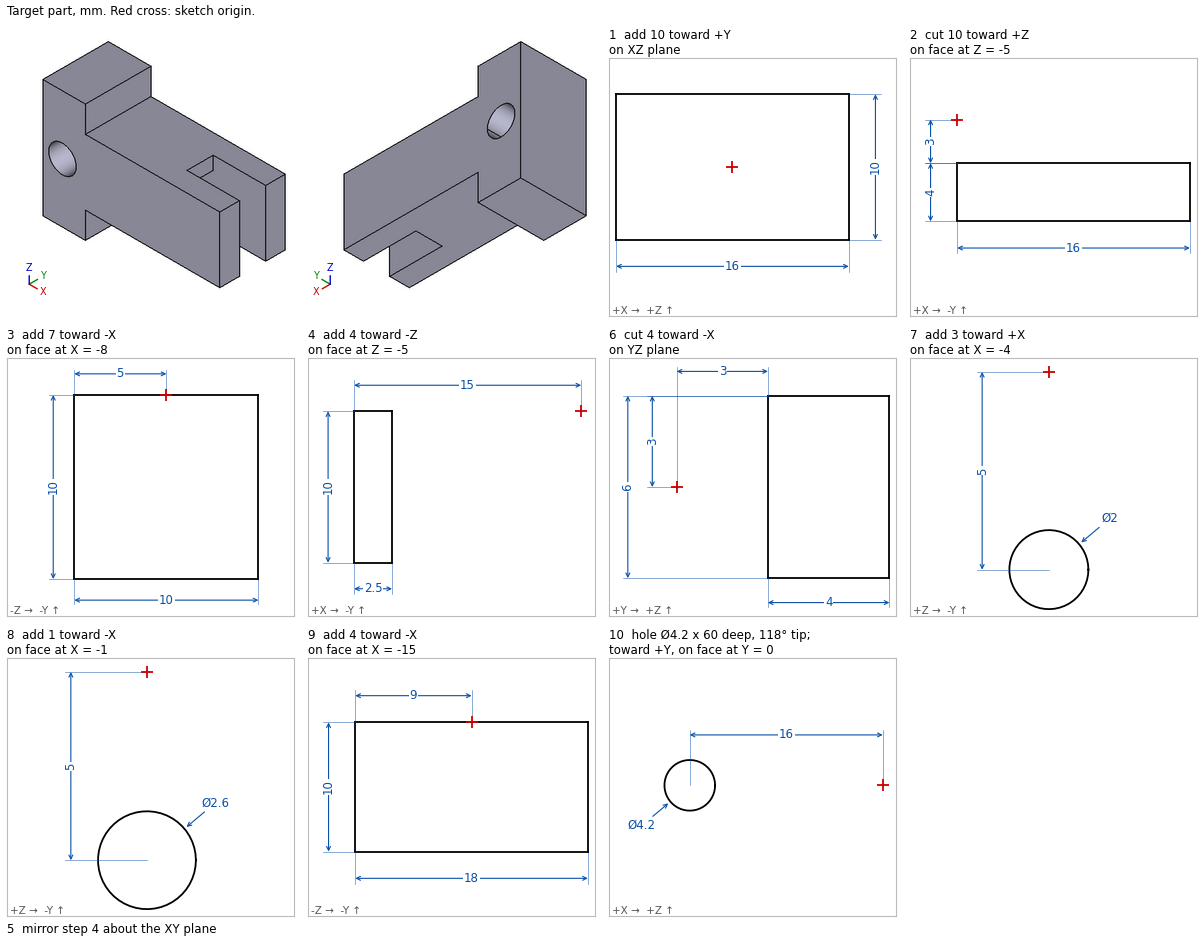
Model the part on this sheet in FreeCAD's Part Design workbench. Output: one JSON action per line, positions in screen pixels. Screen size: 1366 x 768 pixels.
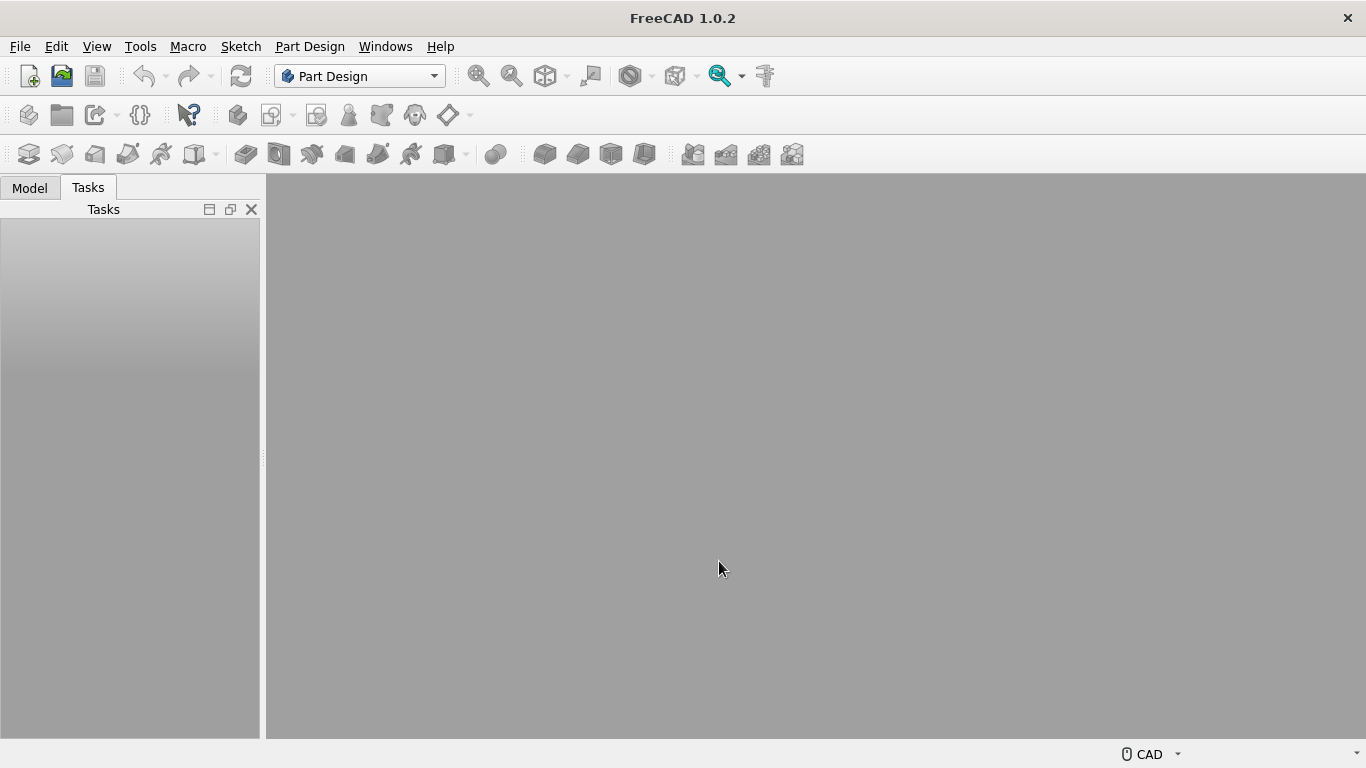
{"action": "left_click", "coordinate": [29, 76]}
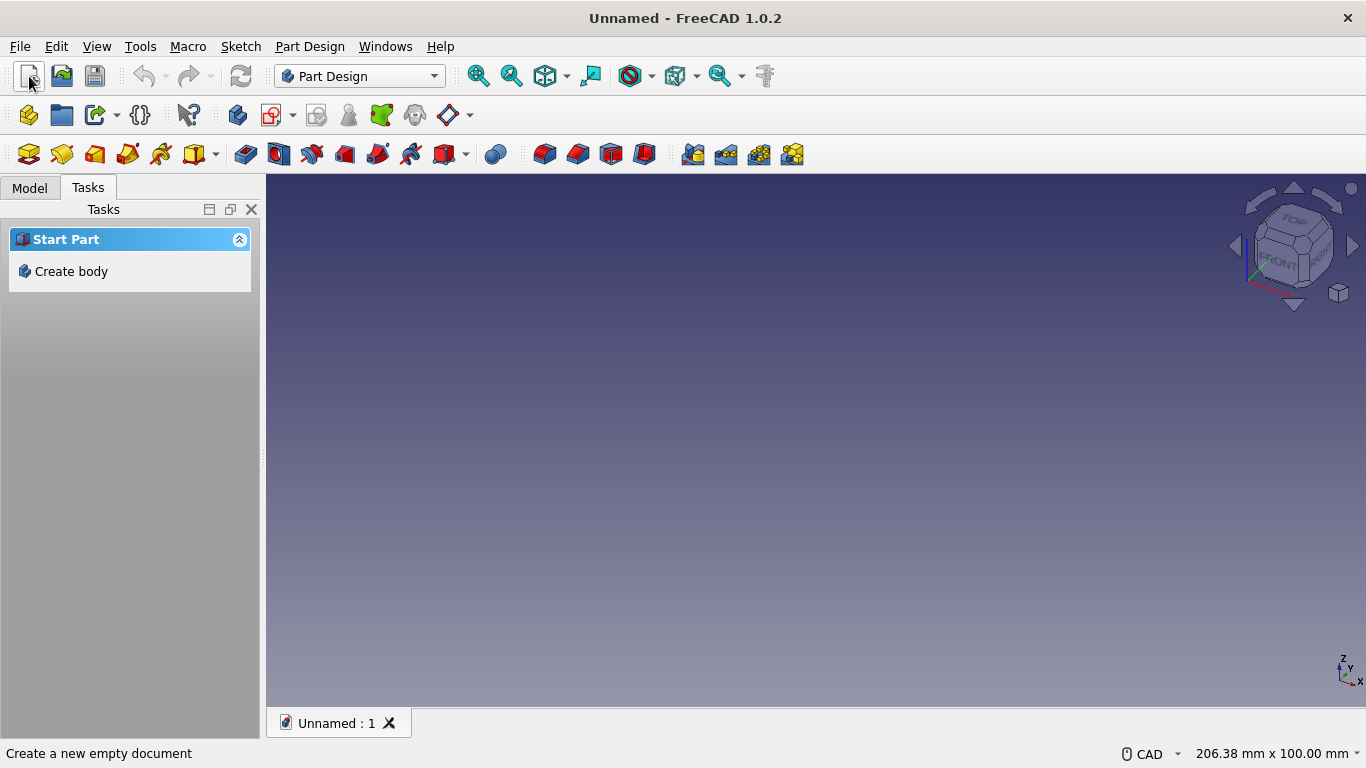
{"action": "left_click", "coordinate": [270, 116]}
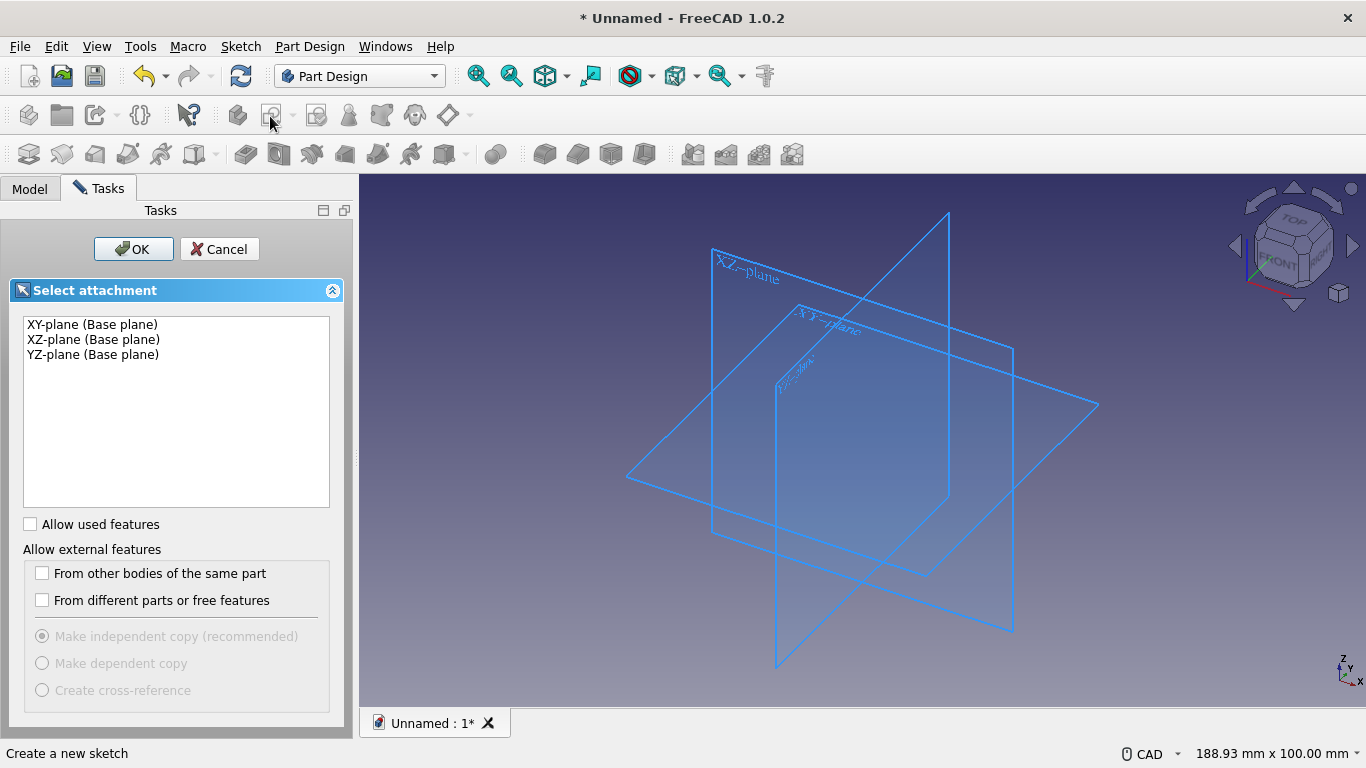
{"action": "left_click", "coordinate": [84, 340]}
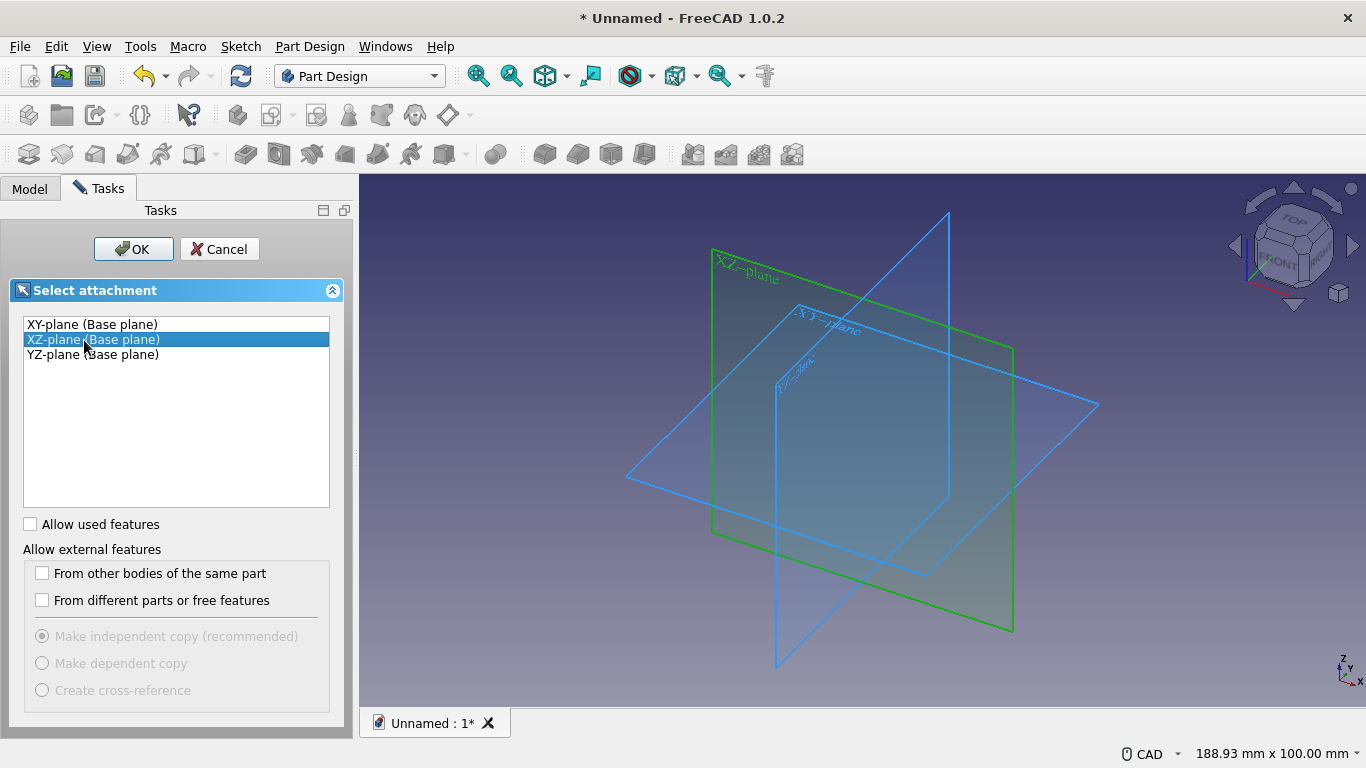
{"action": "left_click", "coordinate": [134, 249]}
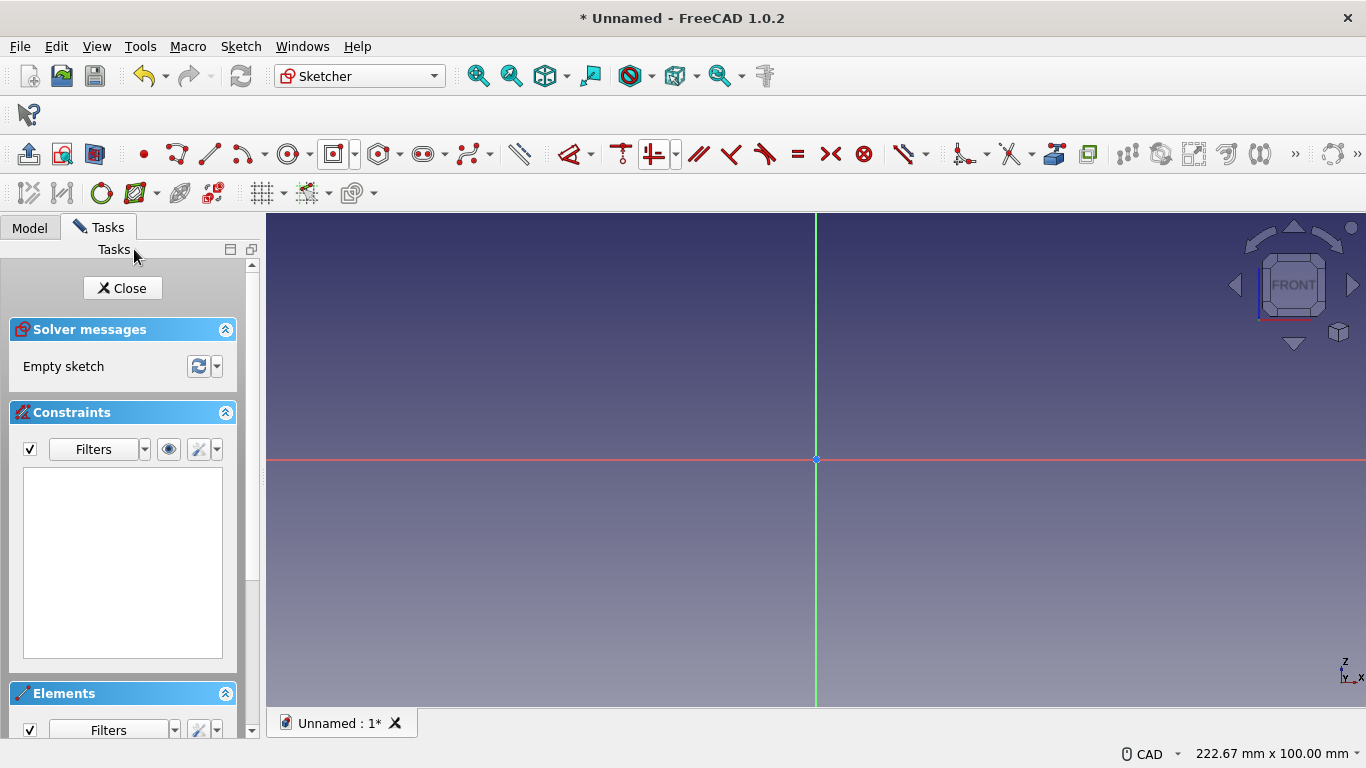
{"action": "scroll", "coordinate": [830, 460], "scroll_direction": "up", "scroll_amount": 9}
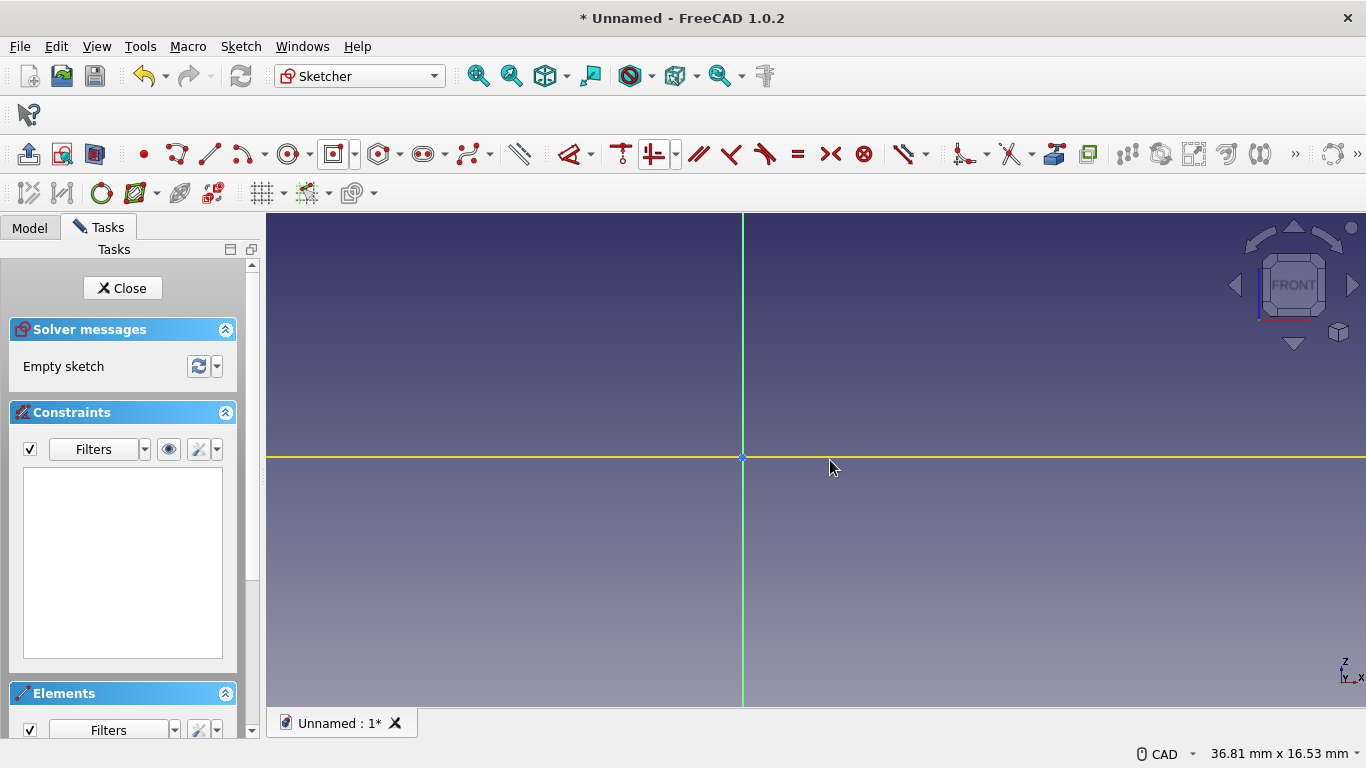
{"action": "left_click", "coordinate": [332, 154]}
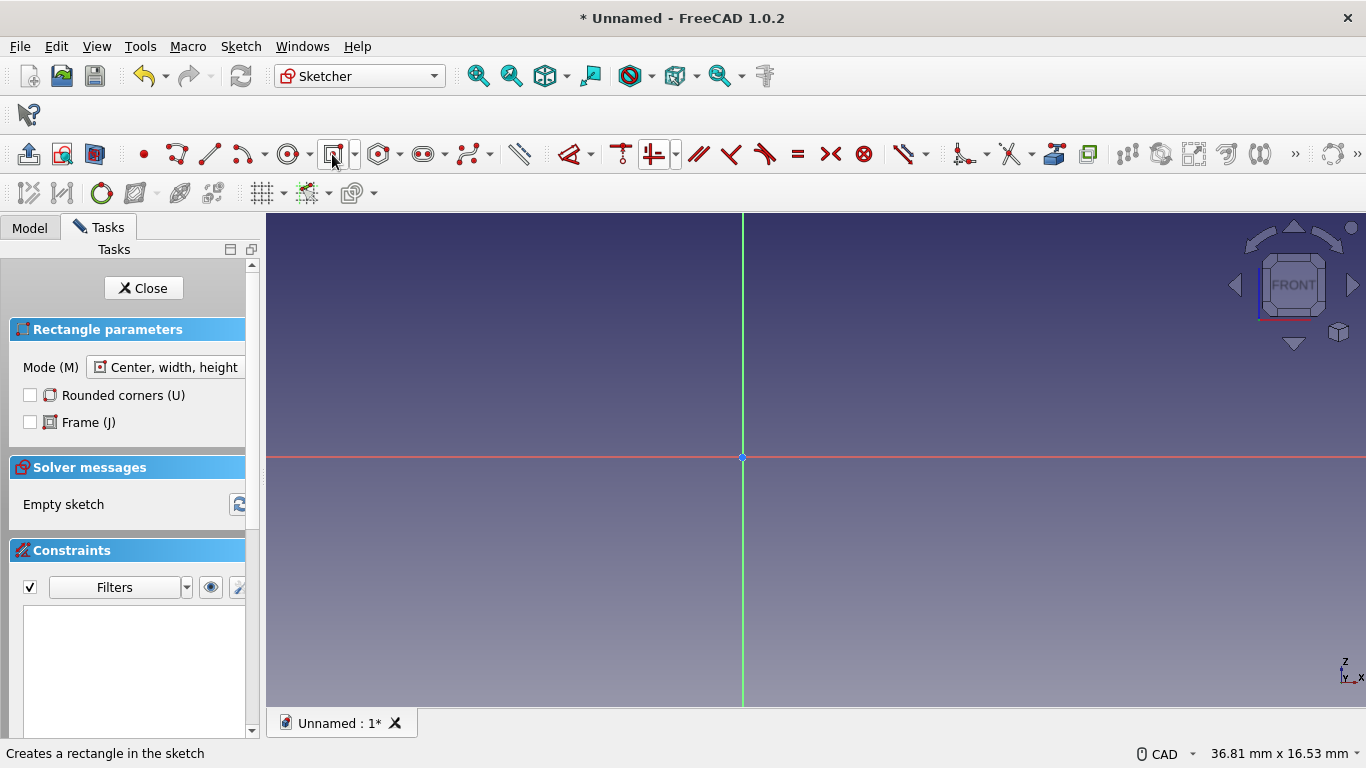
{"action": "left_click", "coordinate": [743, 457]}
{"action": "left_click", "coordinate": [982, 308]}
{"action": "key", "text": "Escape"}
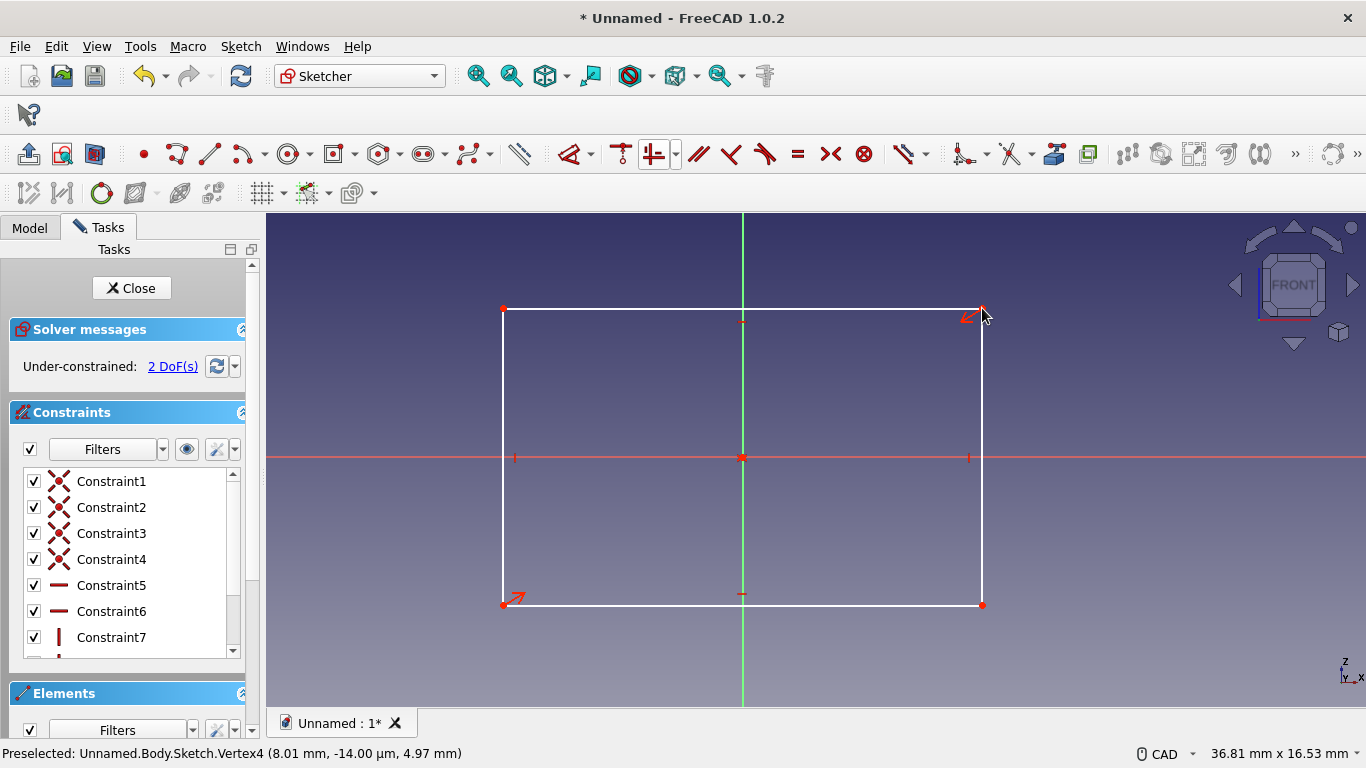
{"action": "left_click", "coordinate": [568, 154]}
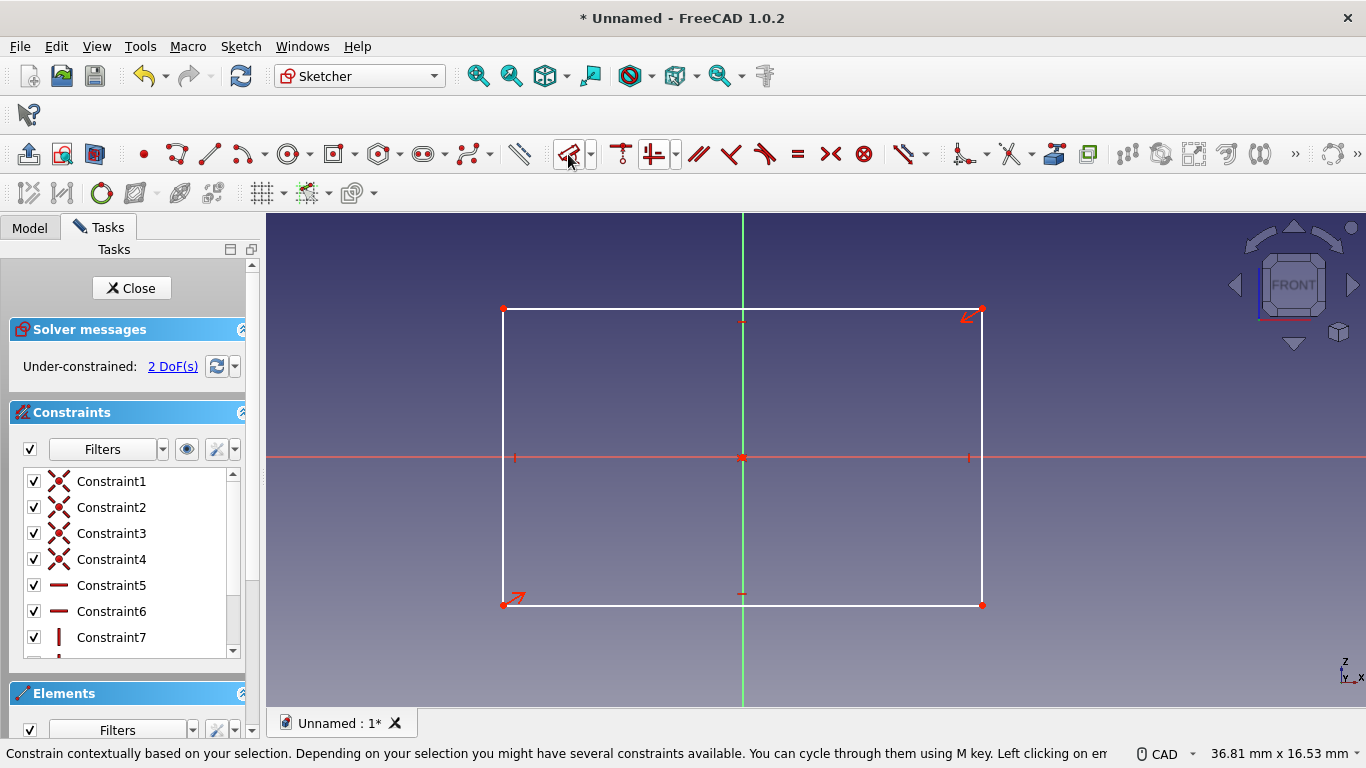
{"action": "left_click", "coordinate": [647, 606]}
{"action": "left_click", "coordinate": [633, 640]}